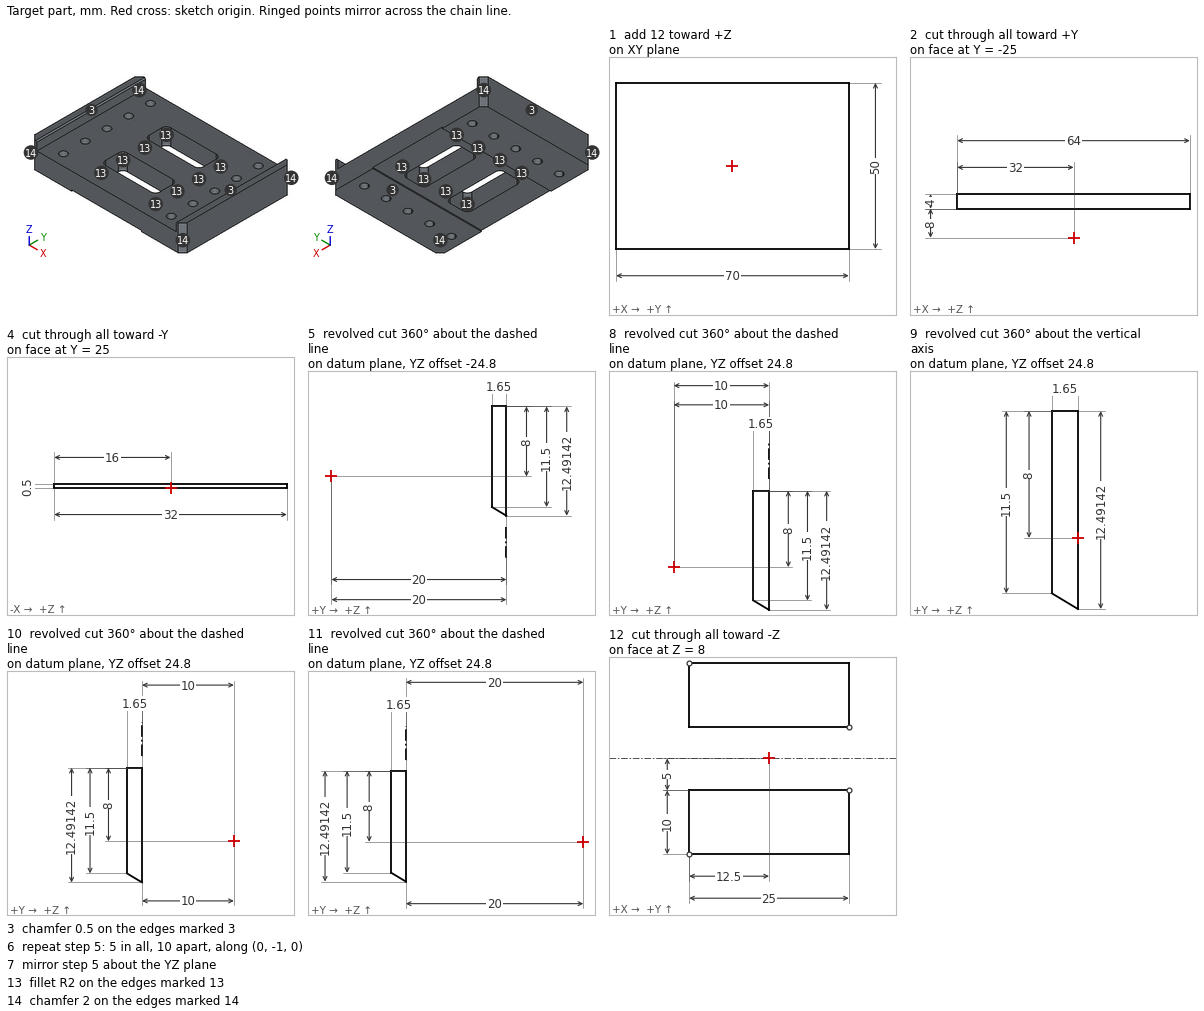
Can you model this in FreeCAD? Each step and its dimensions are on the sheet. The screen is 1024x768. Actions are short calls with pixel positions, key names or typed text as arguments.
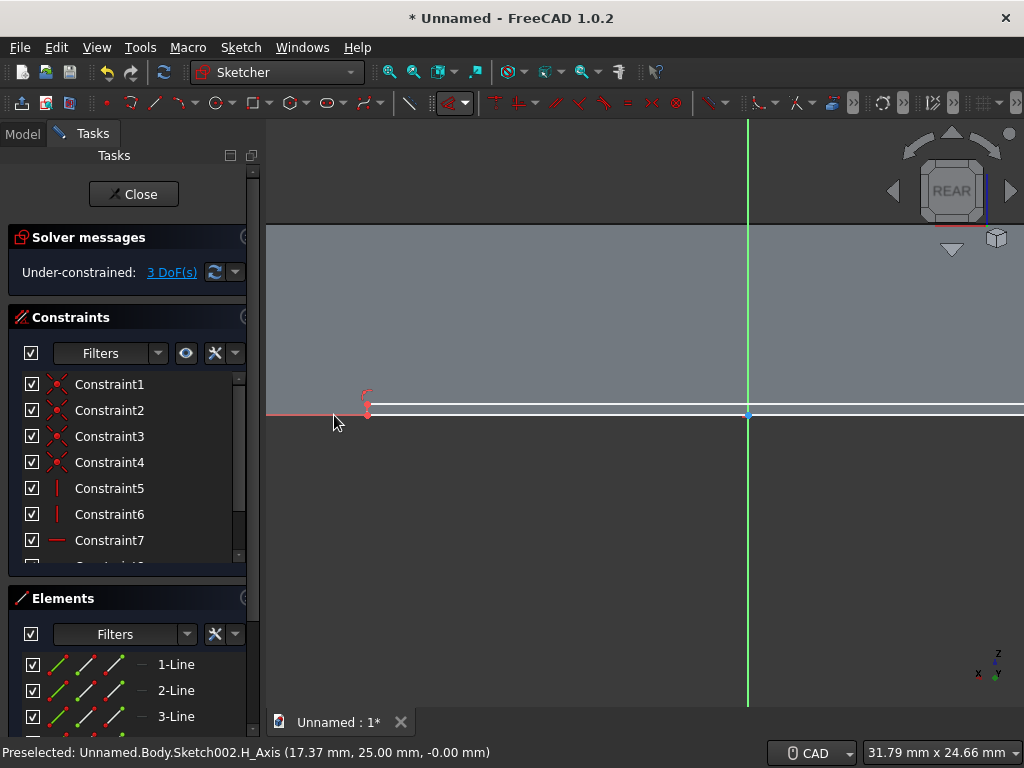
scroll(596, 415, up, 2)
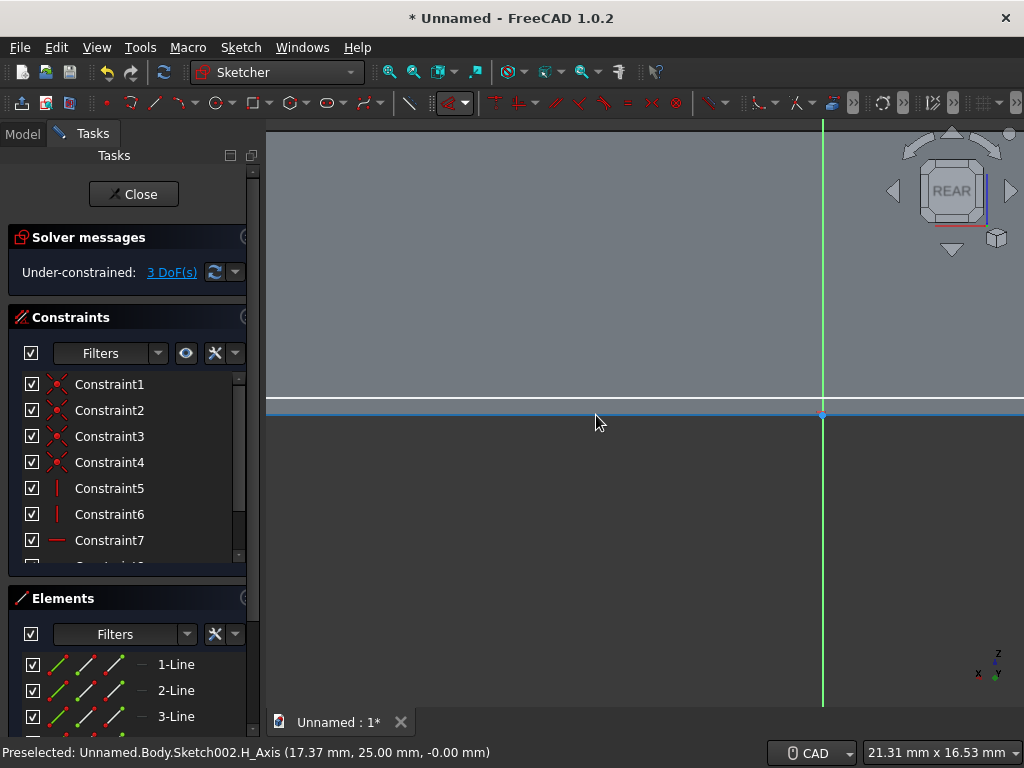
click(596, 415)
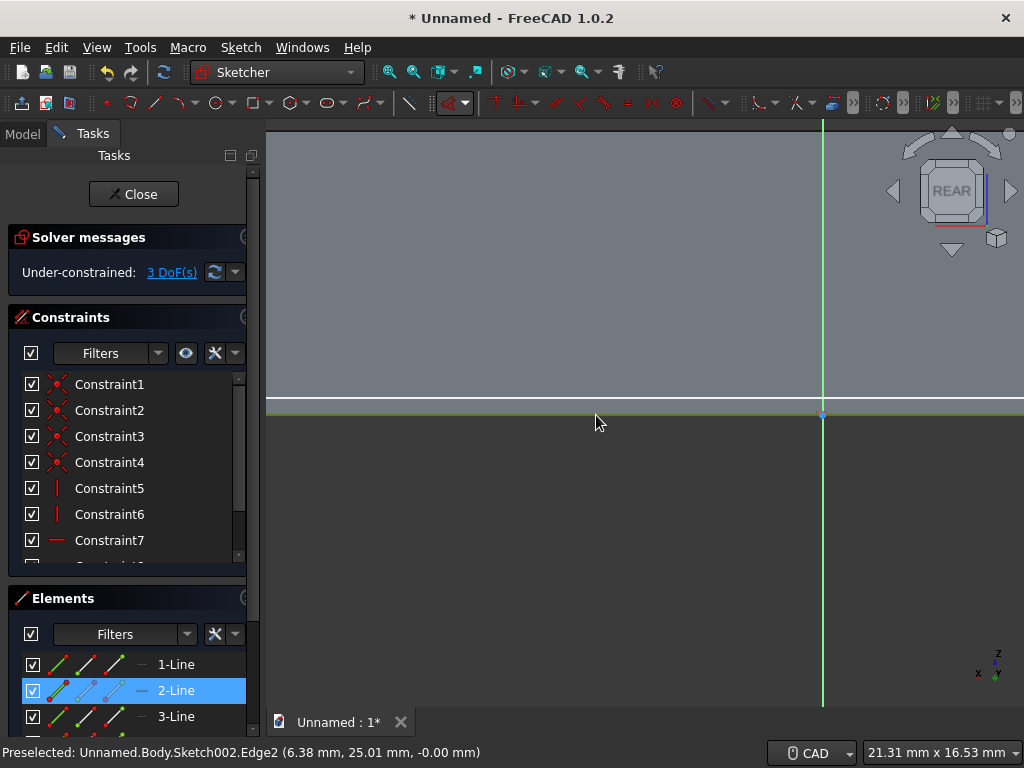
click(468, 104)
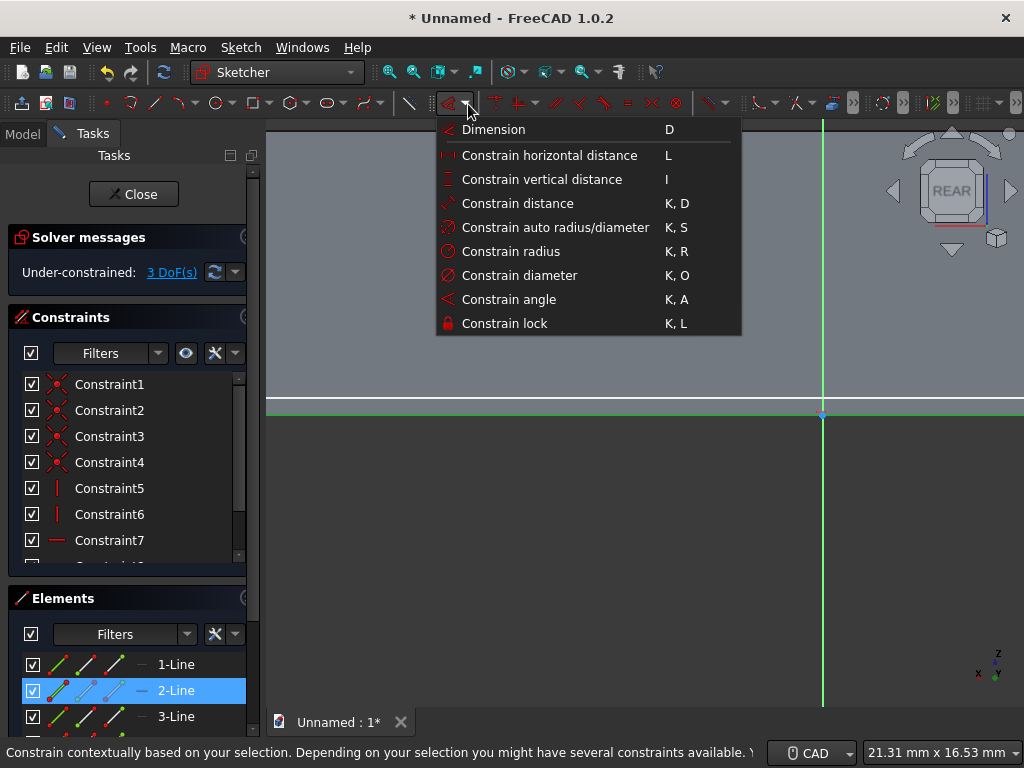
click(589, 155)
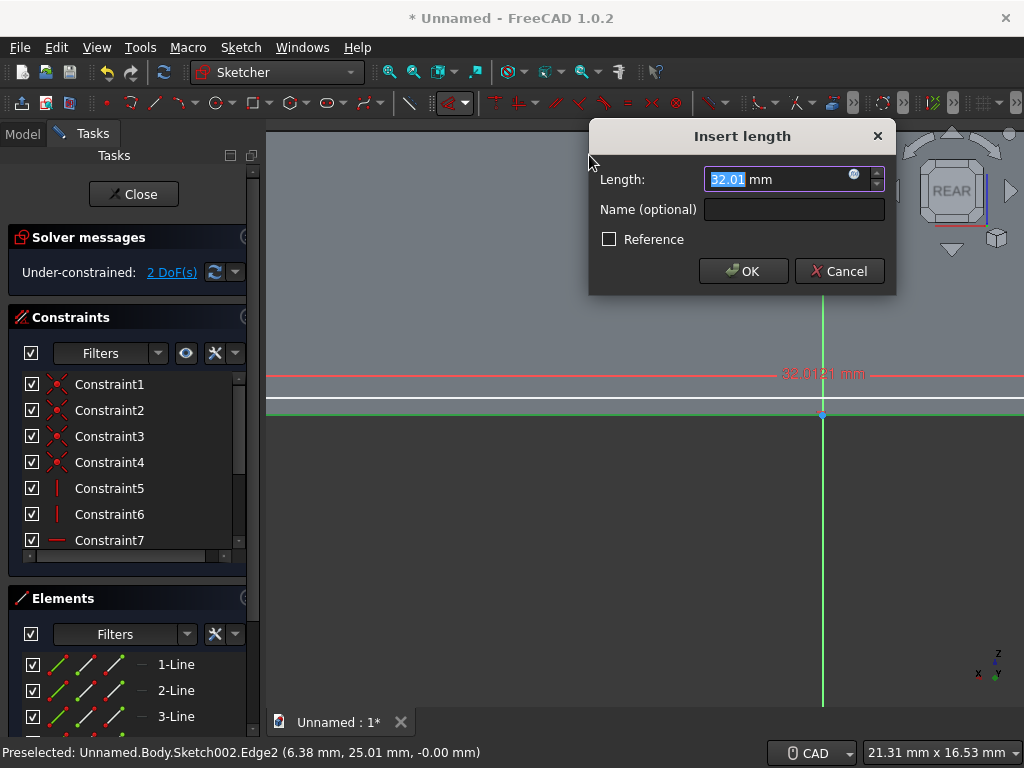
text(32)
key(Return)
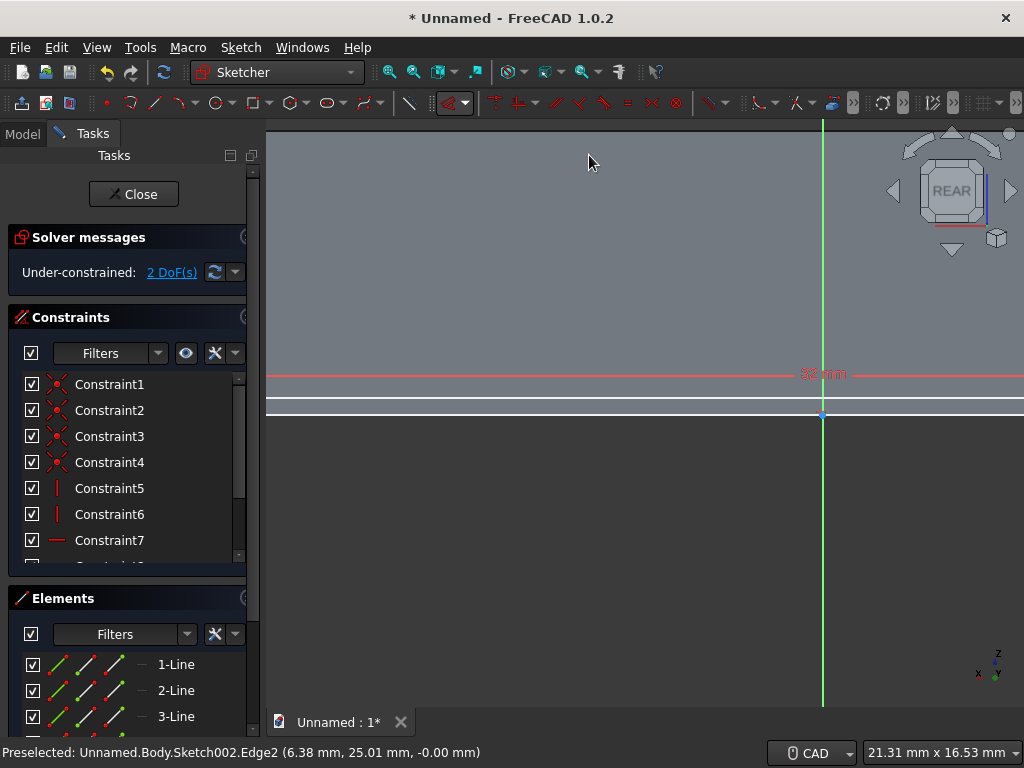
scroll(433, 417, down, 5)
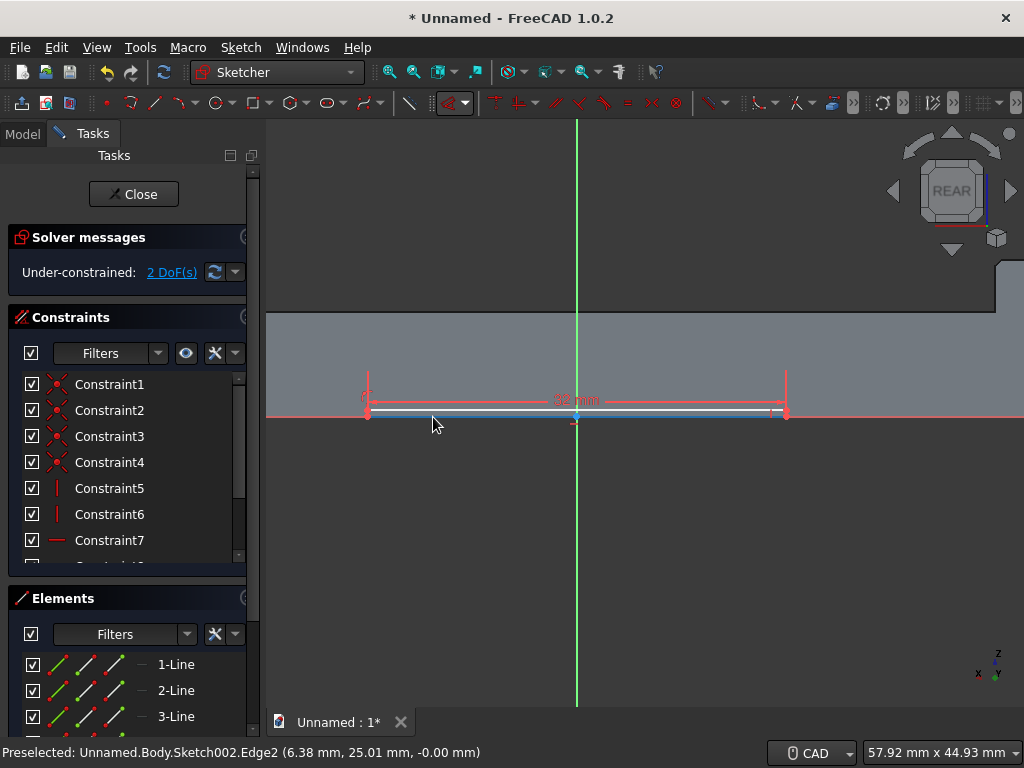
scroll(368, 414, up, 10)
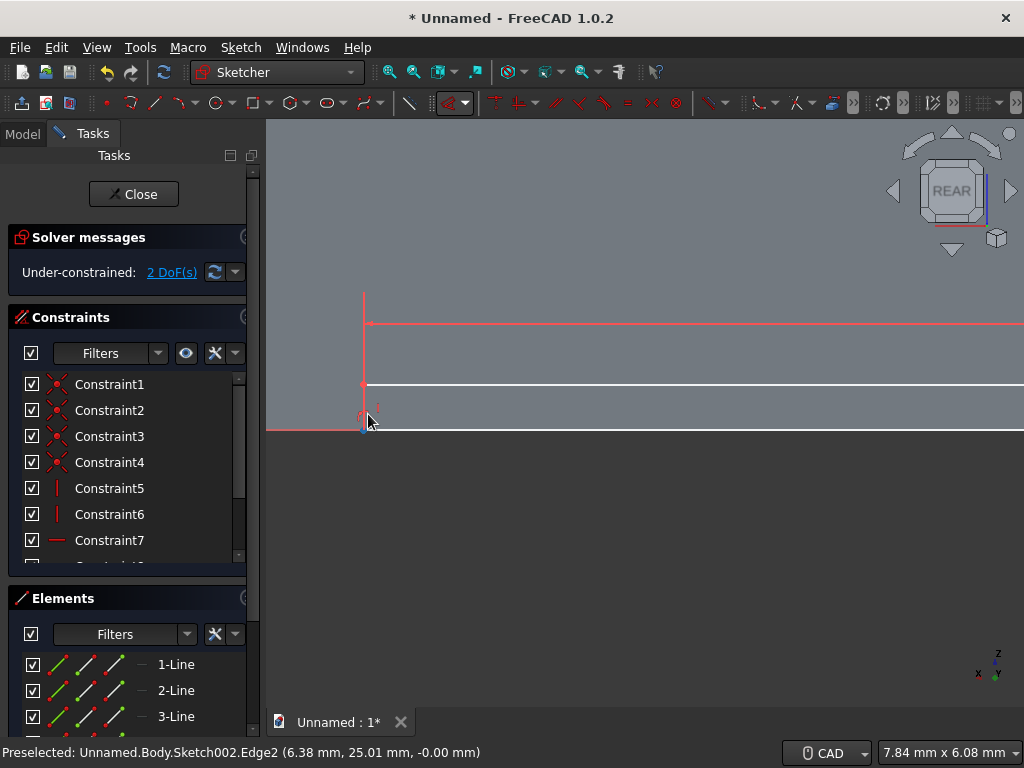
click(364, 407)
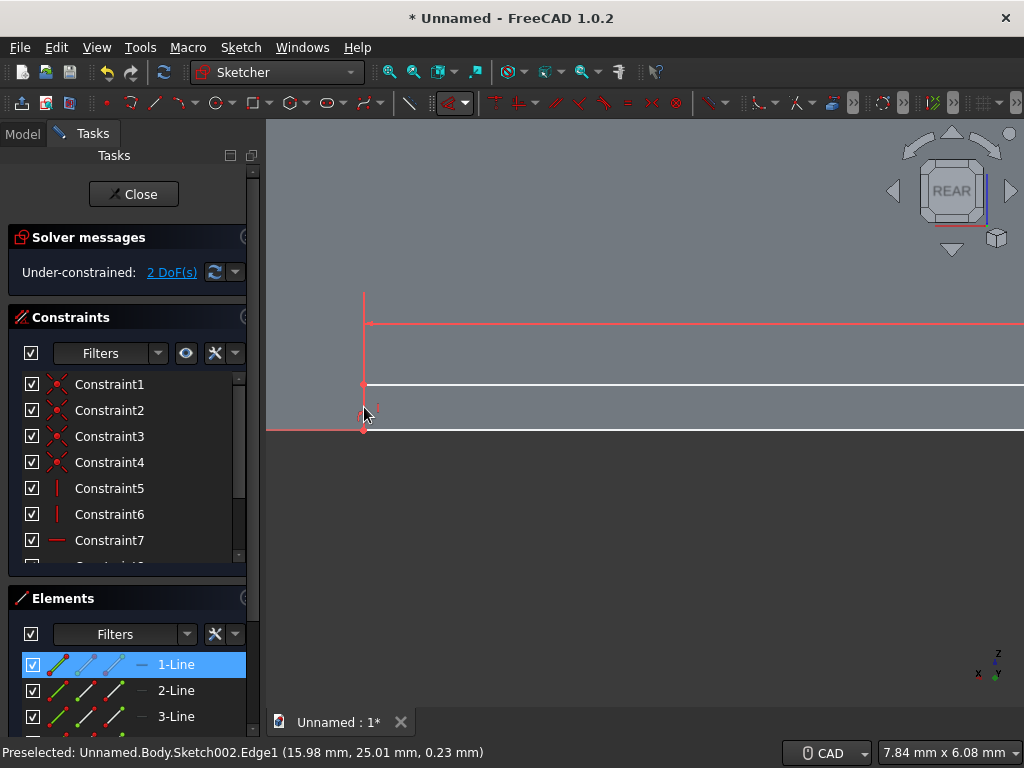
key(i)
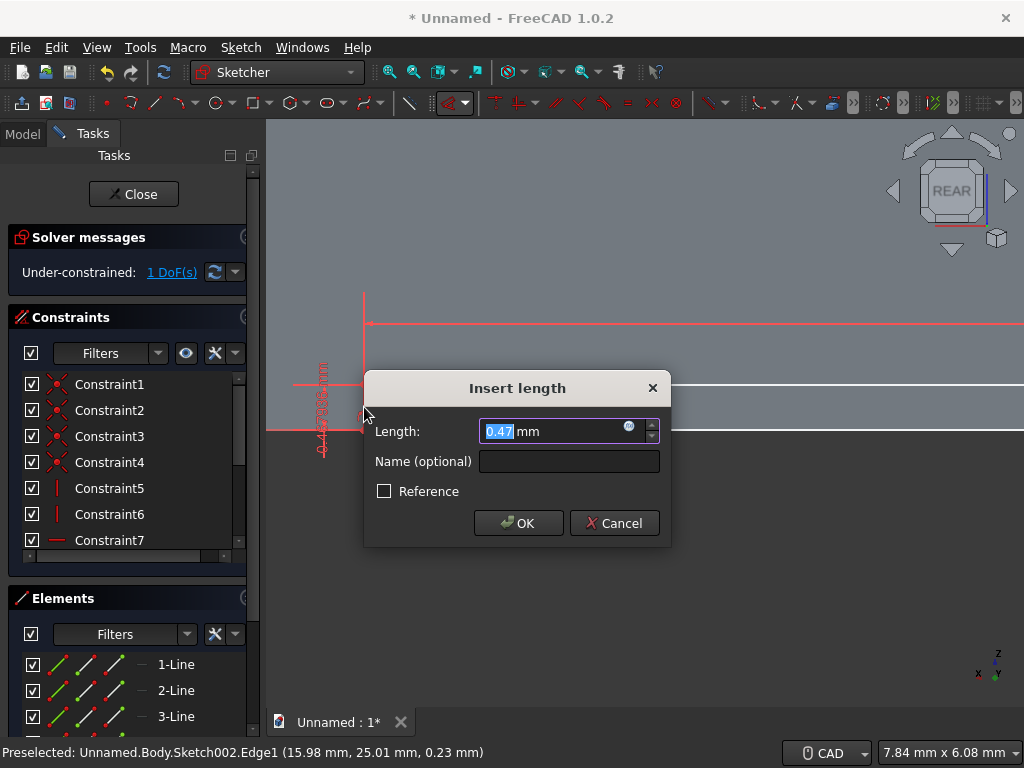
text(0.5)
key(Return)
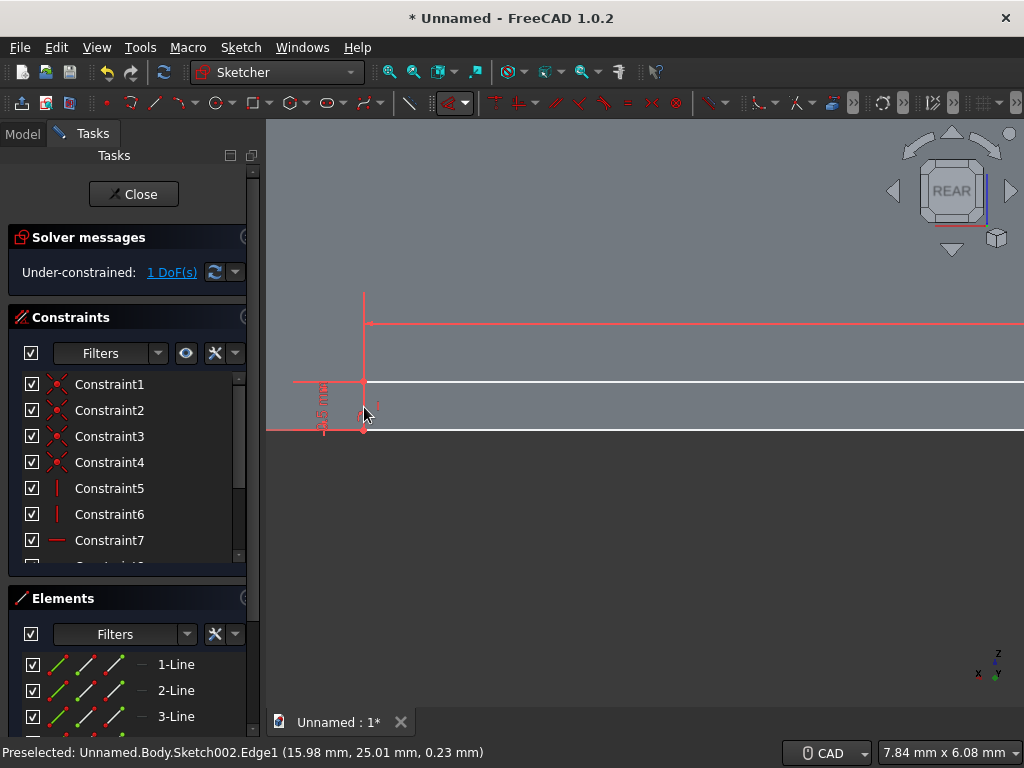
scroll(368, 414, down, 10)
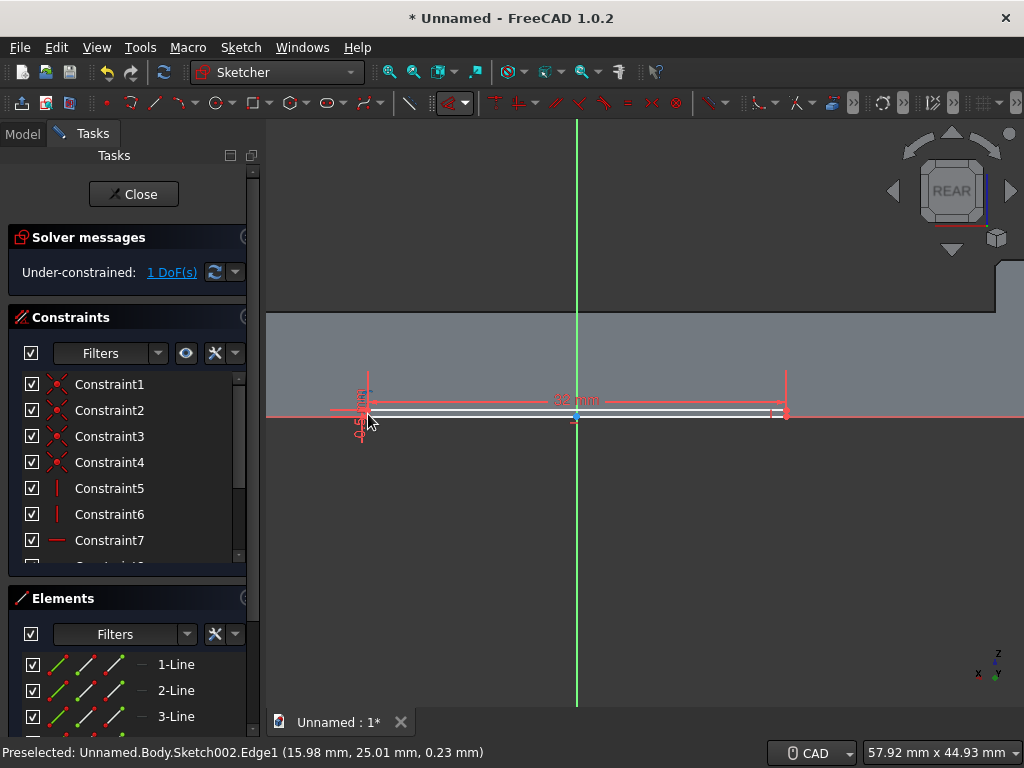
scroll(368, 410, up, 4)